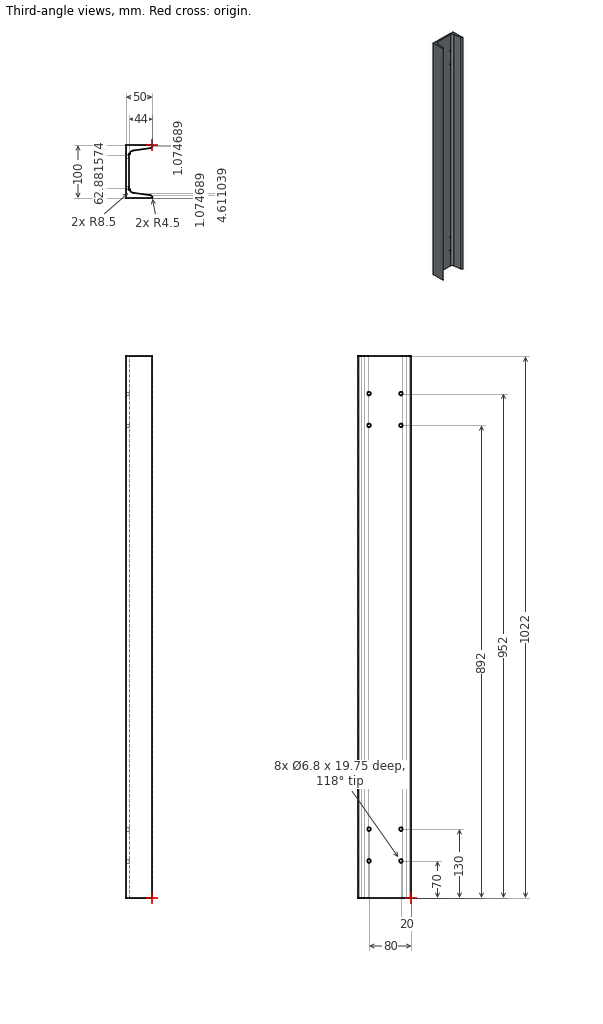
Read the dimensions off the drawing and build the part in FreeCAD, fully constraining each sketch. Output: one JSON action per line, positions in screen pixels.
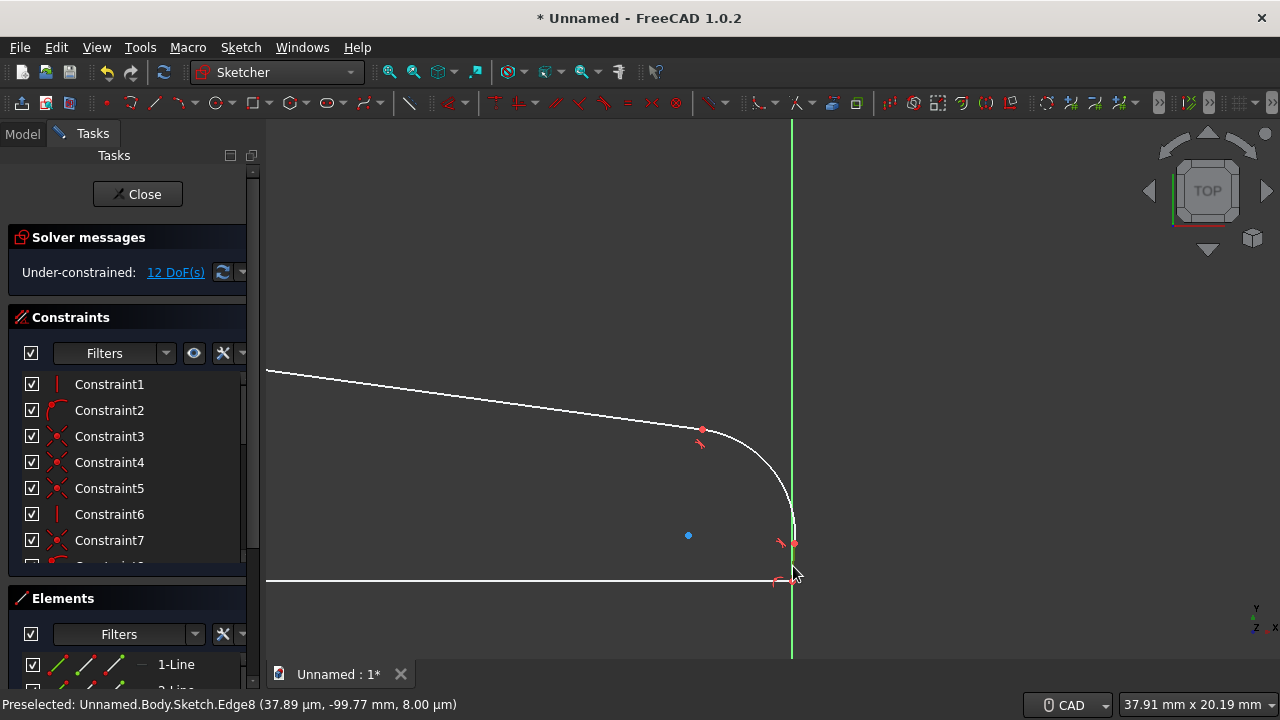
{"action": "left_click", "coordinate": [538, 104]}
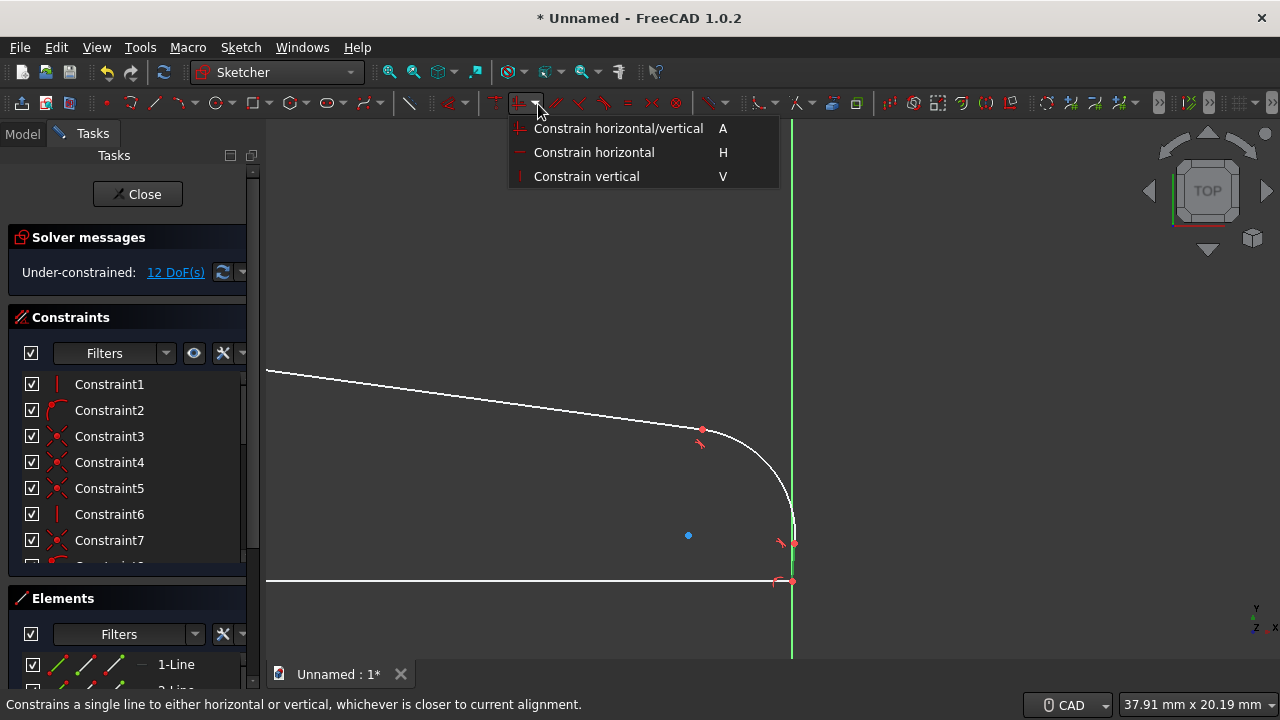
{"action": "left_click", "coordinate": [644, 176]}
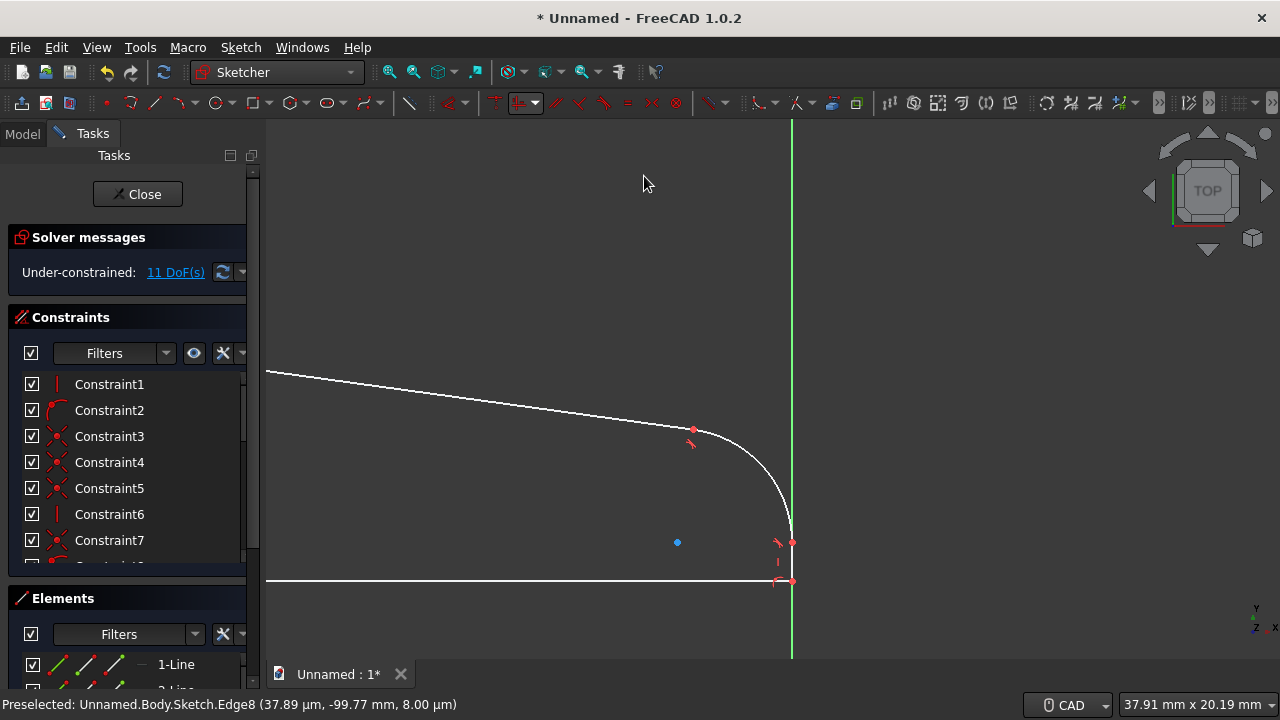
{"action": "scroll", "coordinate": [795, 569], "scroll_direction": "down", "scroll_amount": 10}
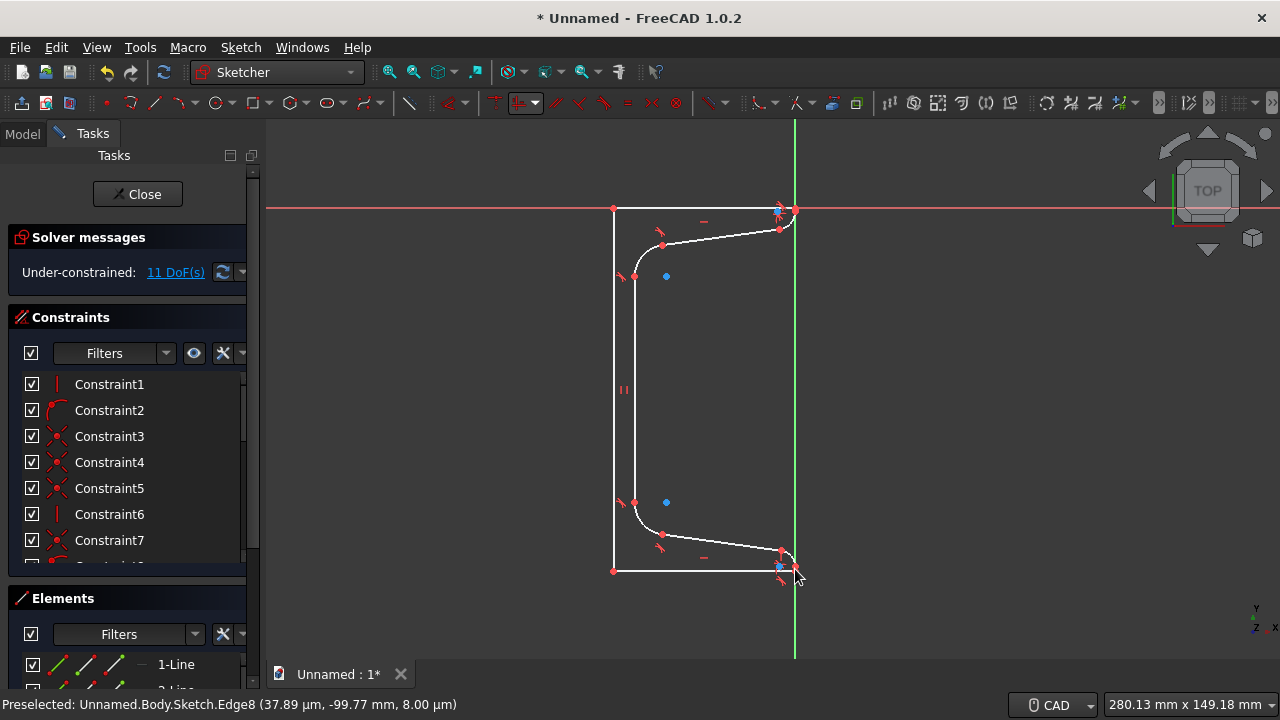
{"action": "left_click", "coordinate": [638, 516]}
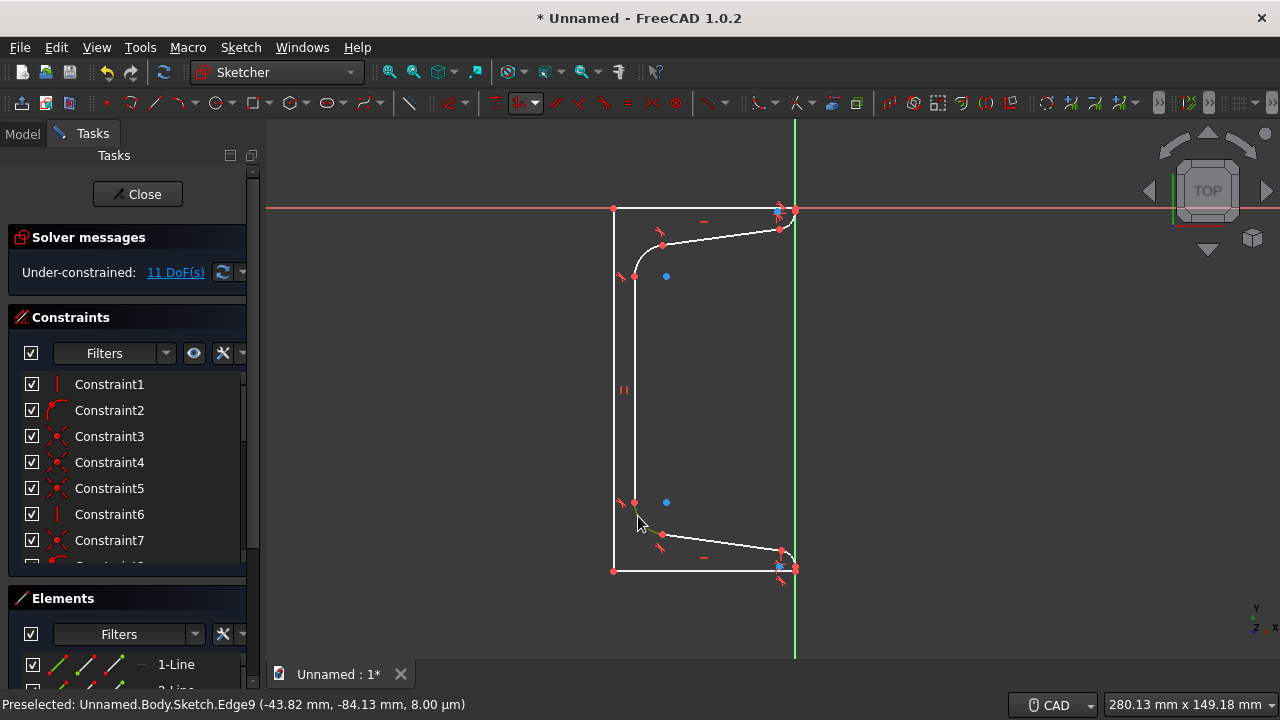
{"action": "left_click", "coordinate": [650, 250]}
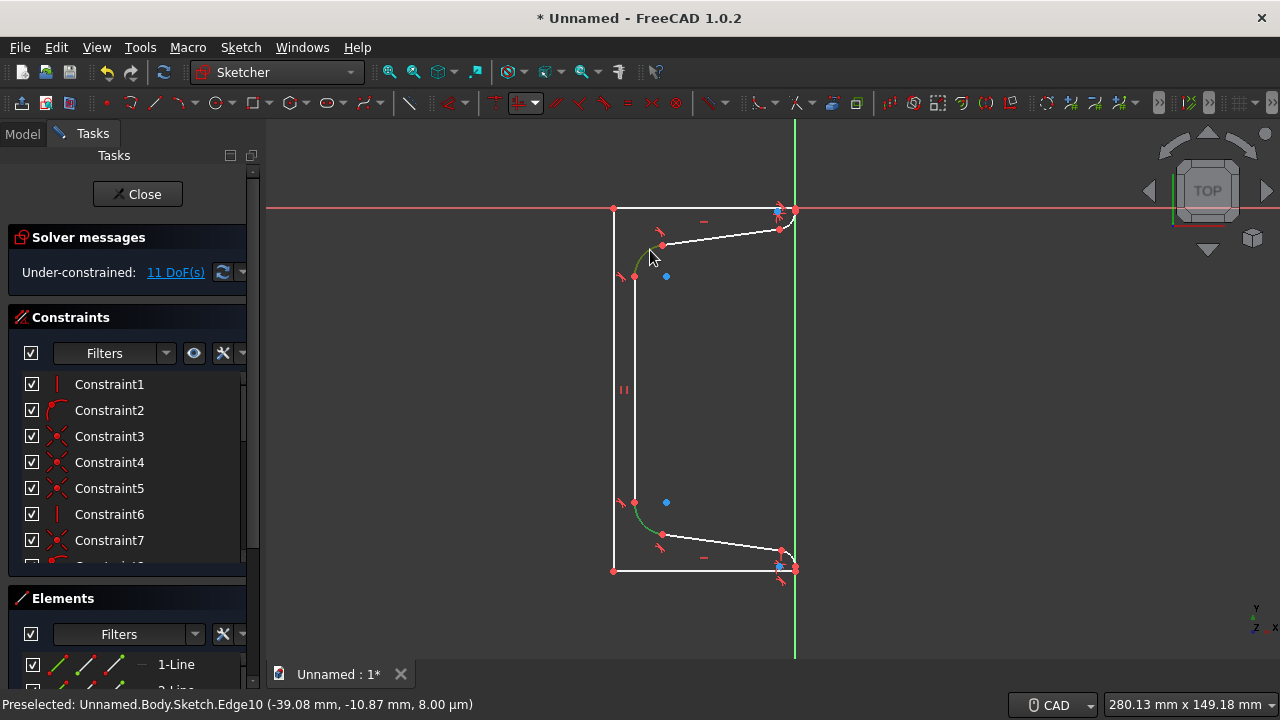
{"action": "left_click", "coordinate": [628, 104]}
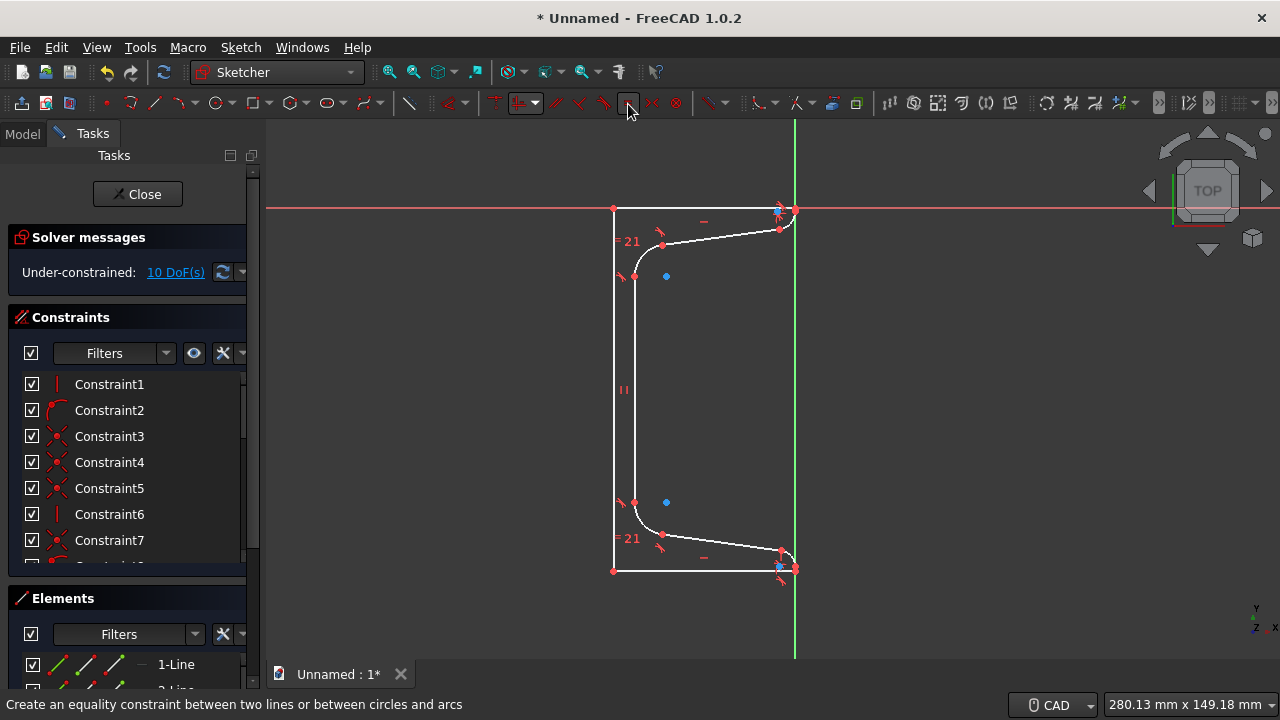
{"action": "scroll", "coordinate": [793, 219], "scroll_direction": "up", "scroll_amount": 4}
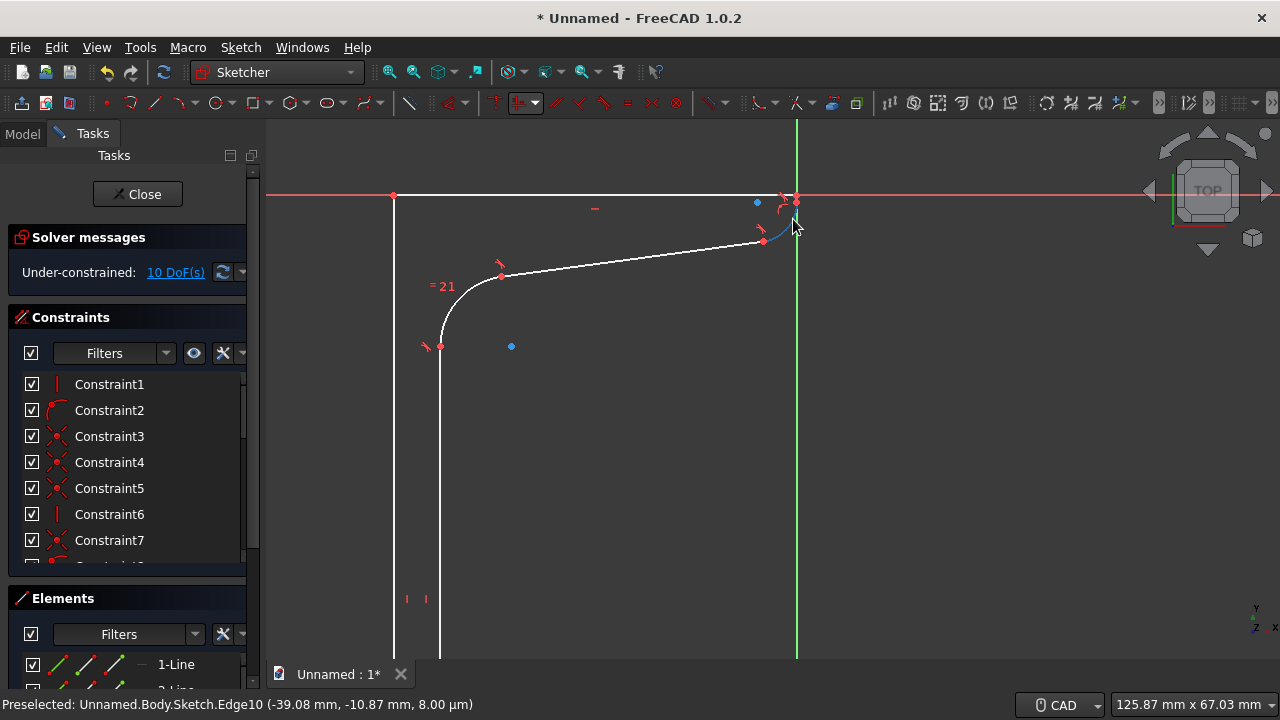
{"action": "left_click", "coordinate": [793, 219]}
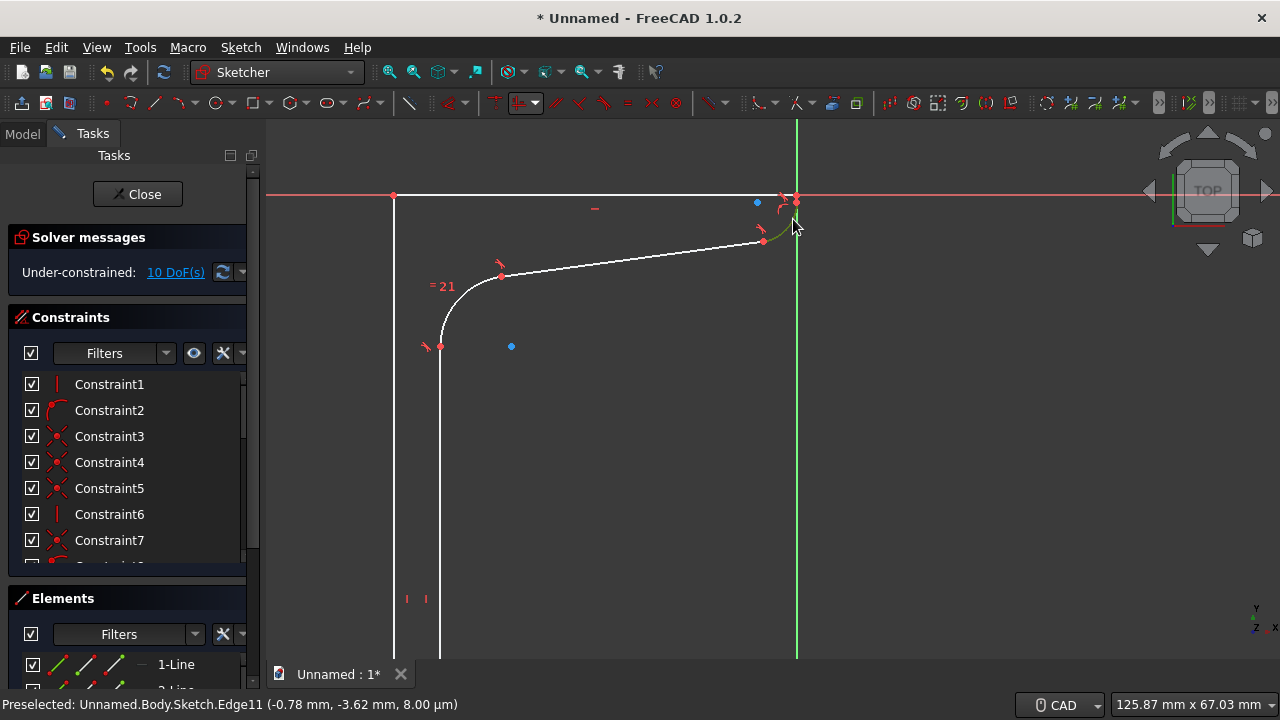
{"action": "scroll", "coordinate": [793, 219], "scroll_direction": "down", "scroll_amount": 4}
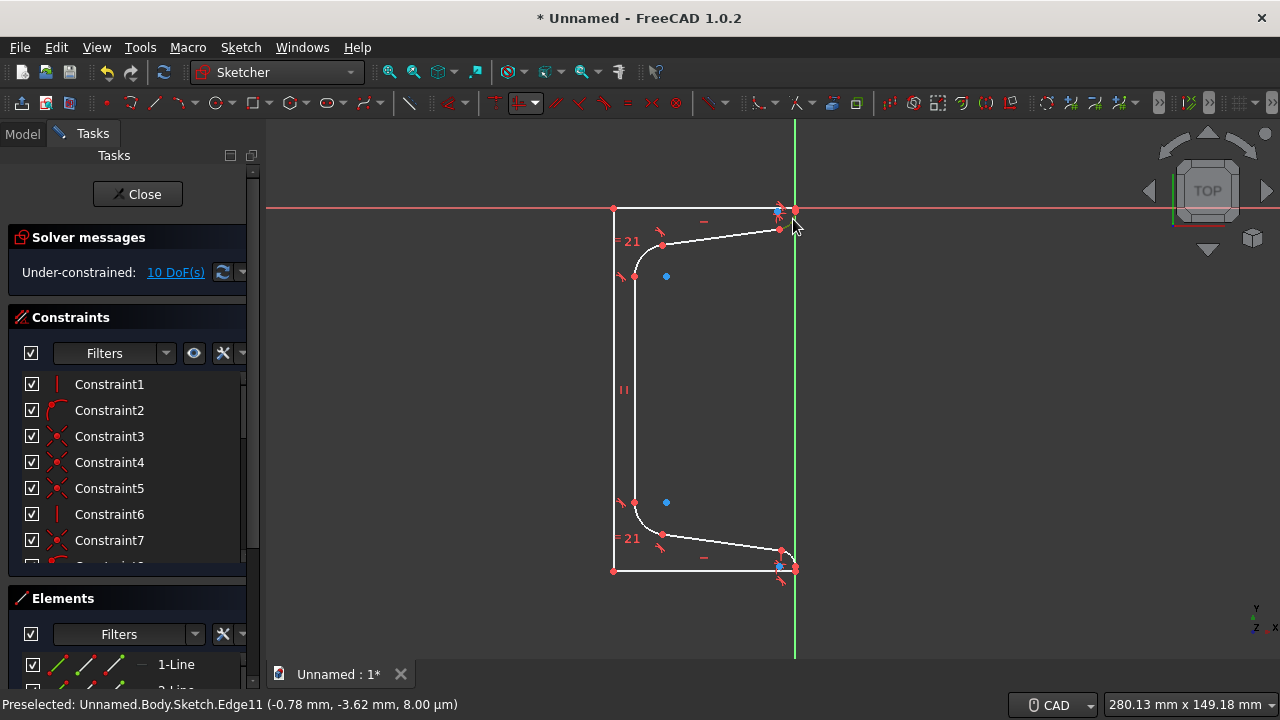
{"action": "scroll", "coordinate": [794, 560], "scroll_direction": "up", "scroll_amount": 4}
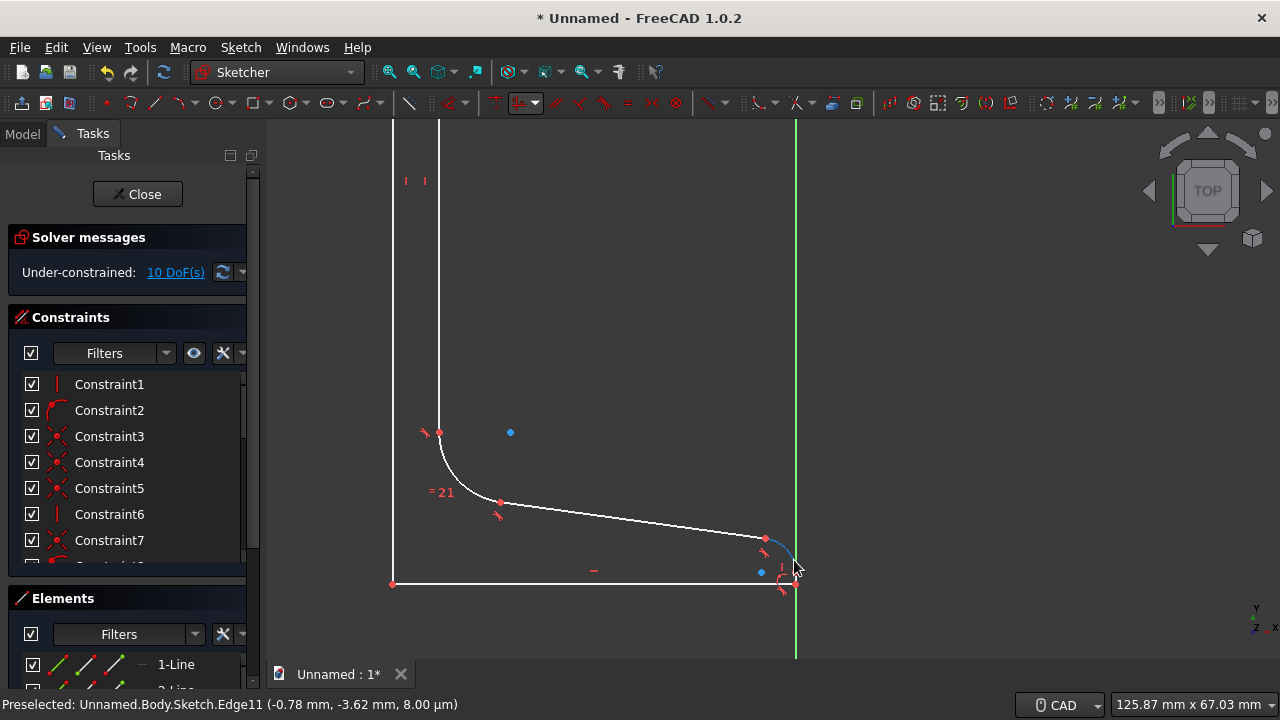
{"action": "left_click", "coordinate": [793, 558]}